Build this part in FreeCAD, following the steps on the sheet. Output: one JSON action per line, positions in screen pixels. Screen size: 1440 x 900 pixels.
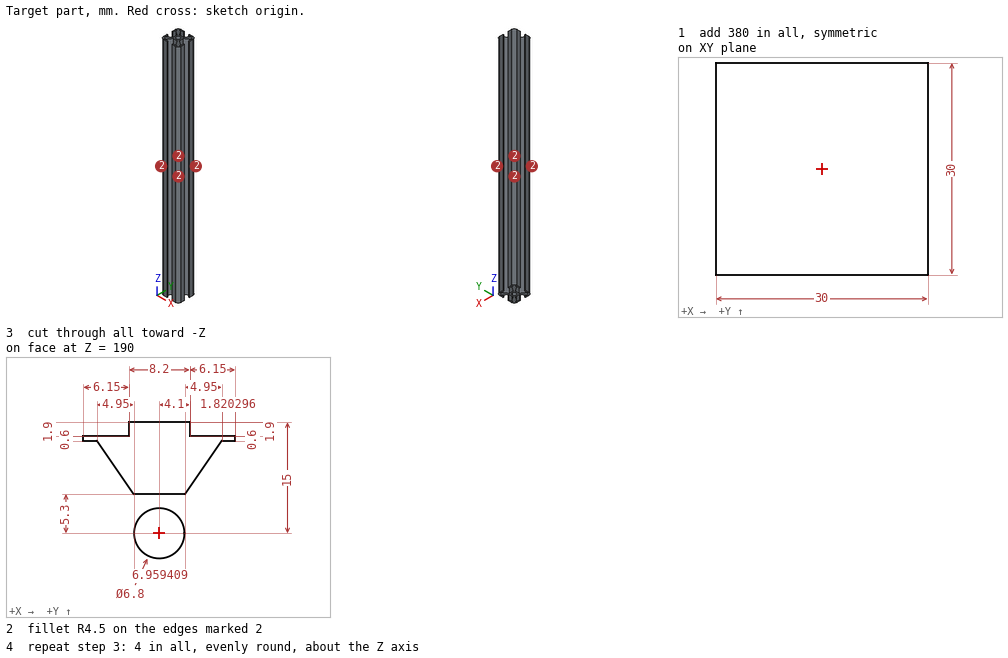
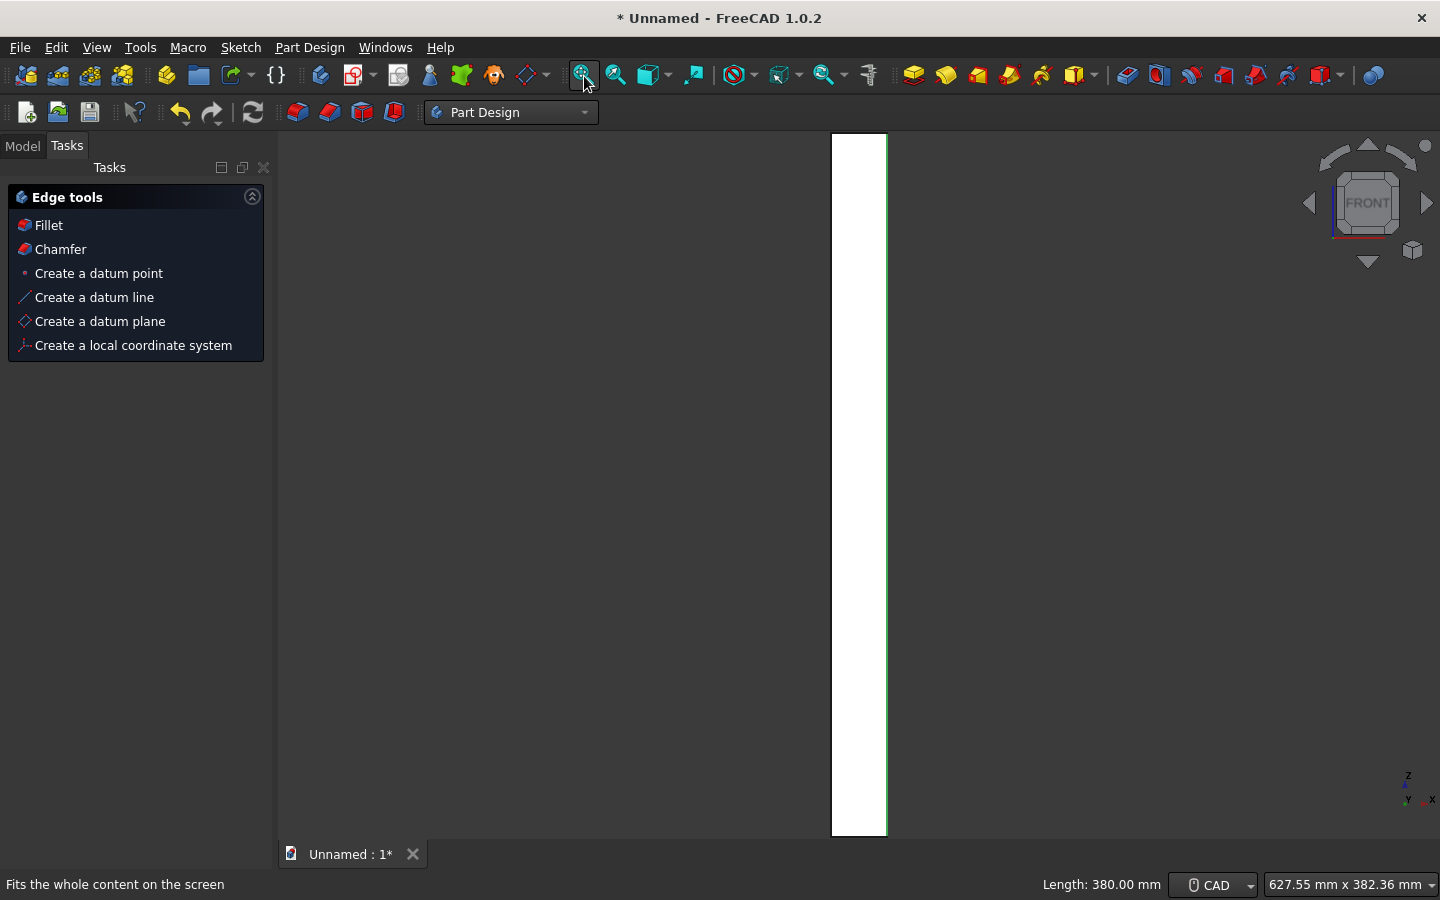
{"action": "left_click", "coordinate": [831, 484], "text": "ctrl"}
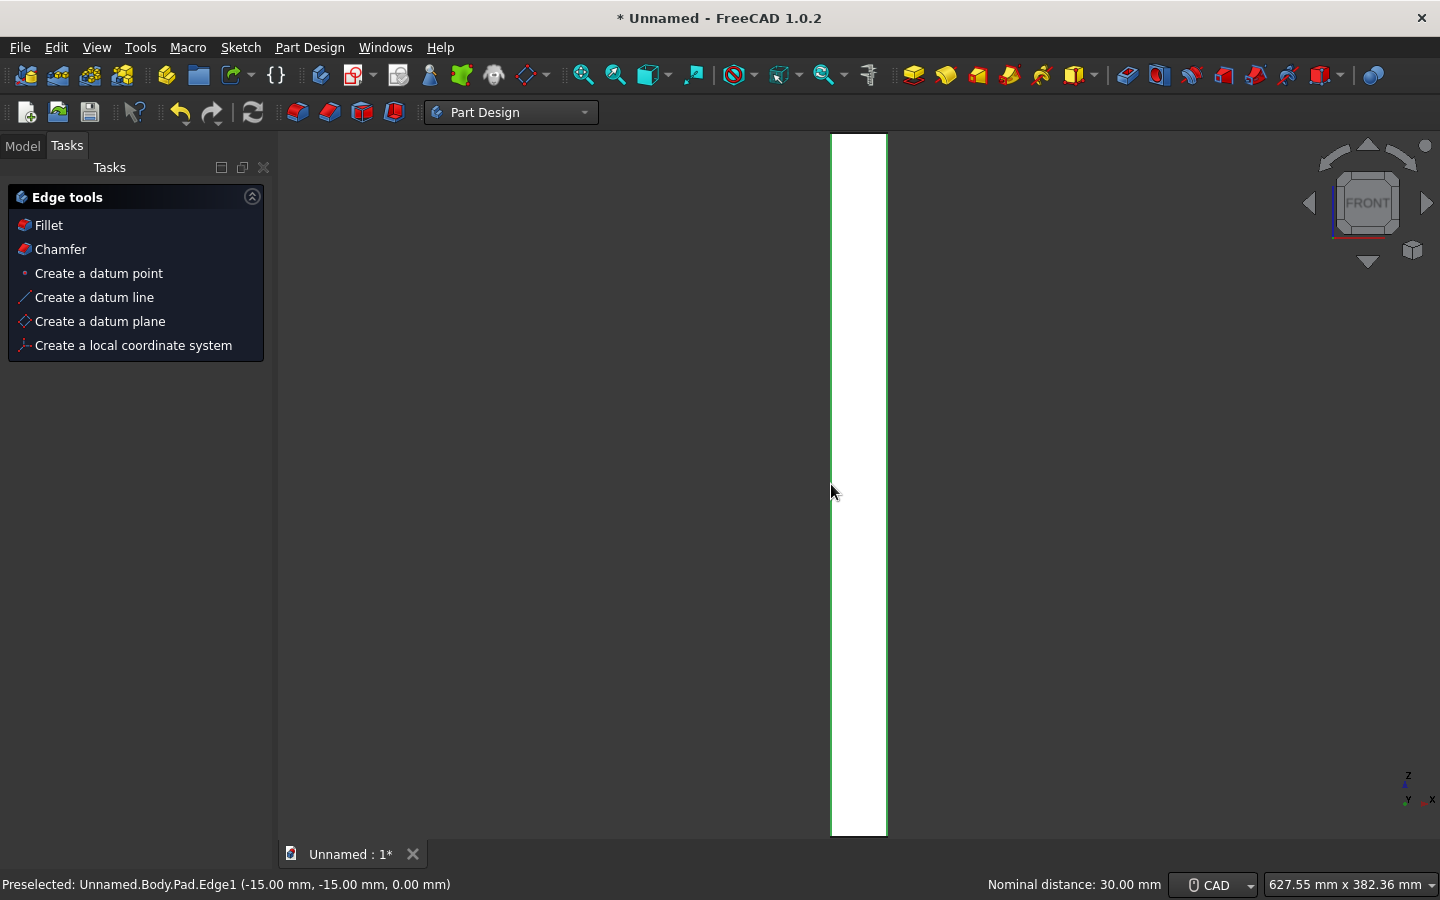
{"action": "key", "text": "3"}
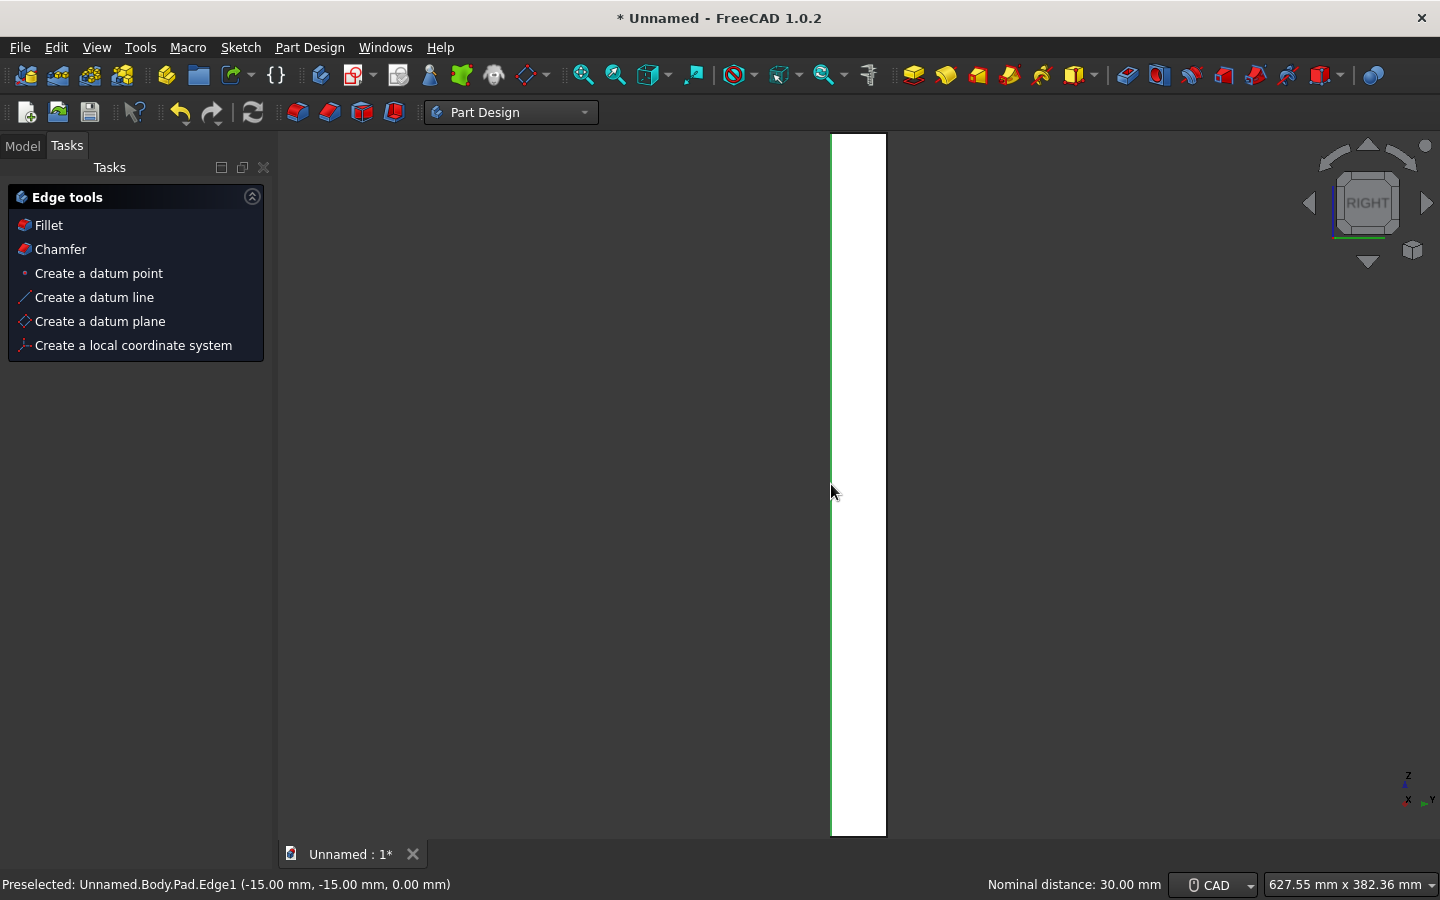
{"action": "left_click", "coordinate": [887, 484], "text": "ctrl"}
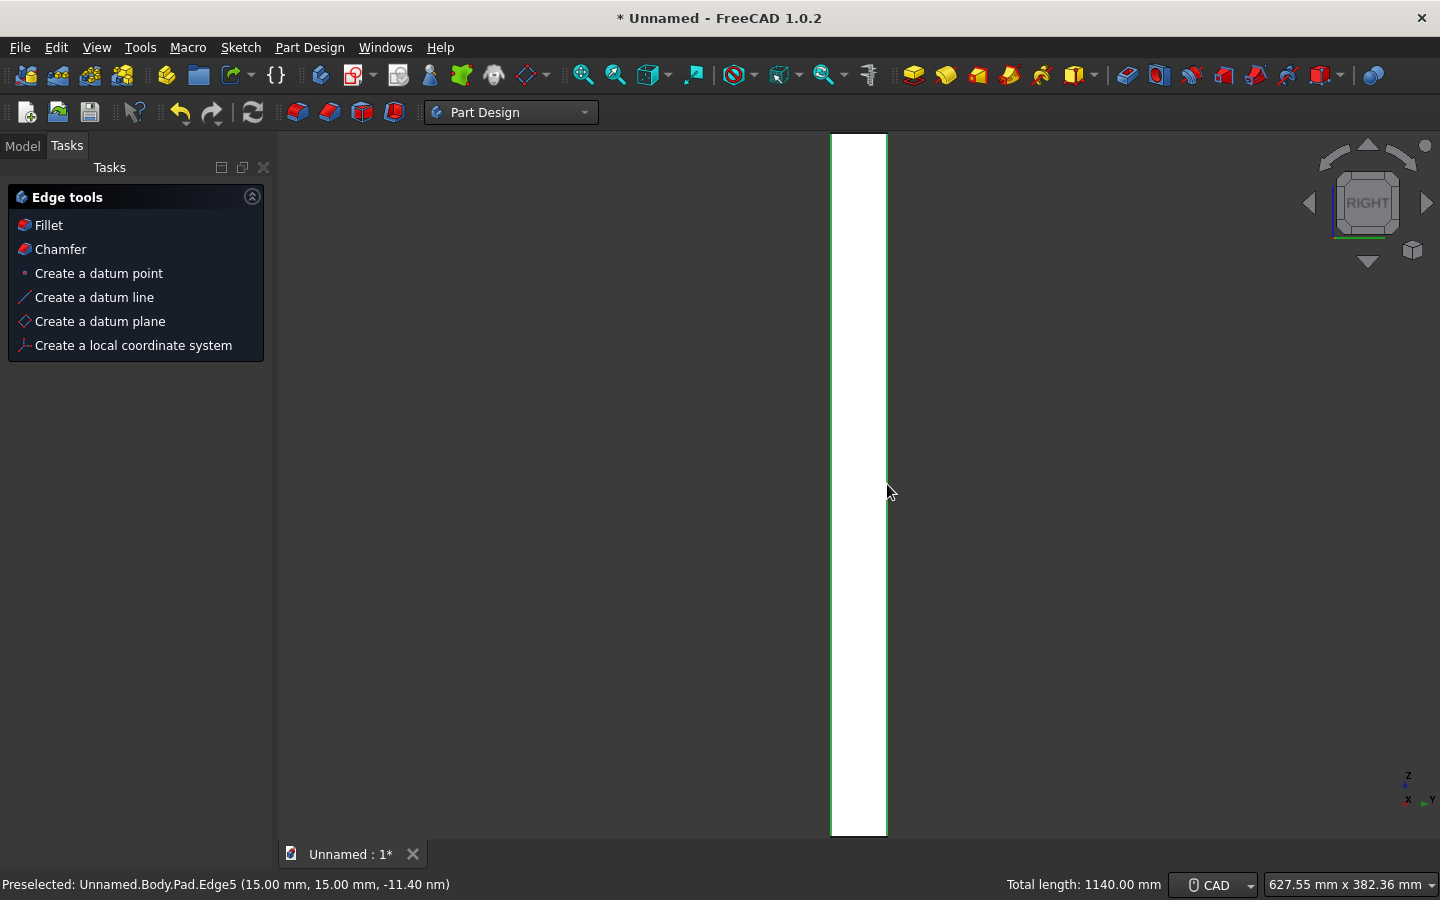
{"action": "key", "text": "5"}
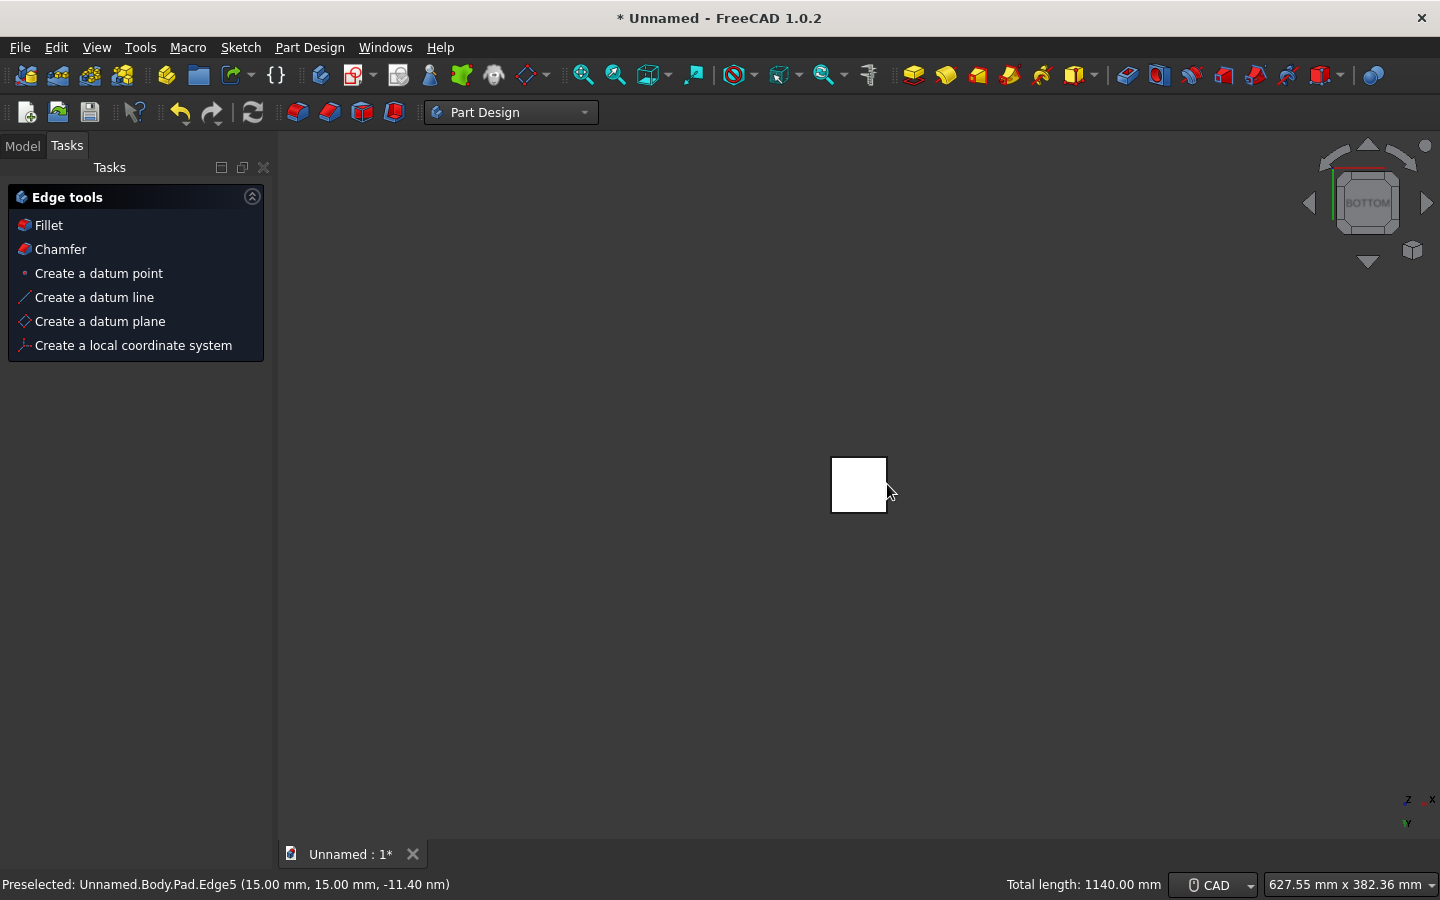
{"action": "left_click", "coordinate": [584, 76]}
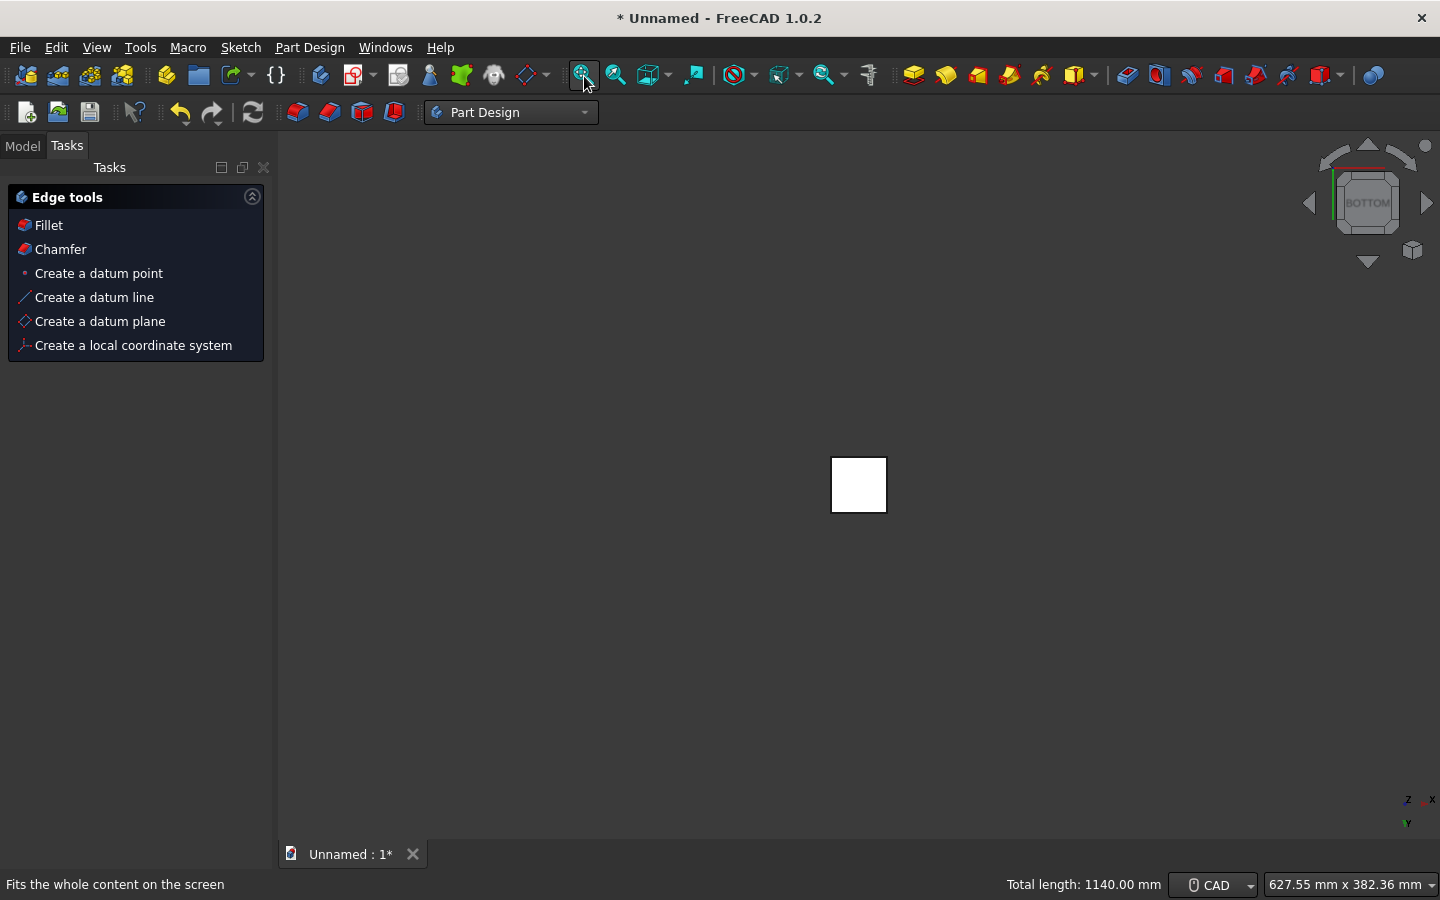
{"action": "key", "text": "4"}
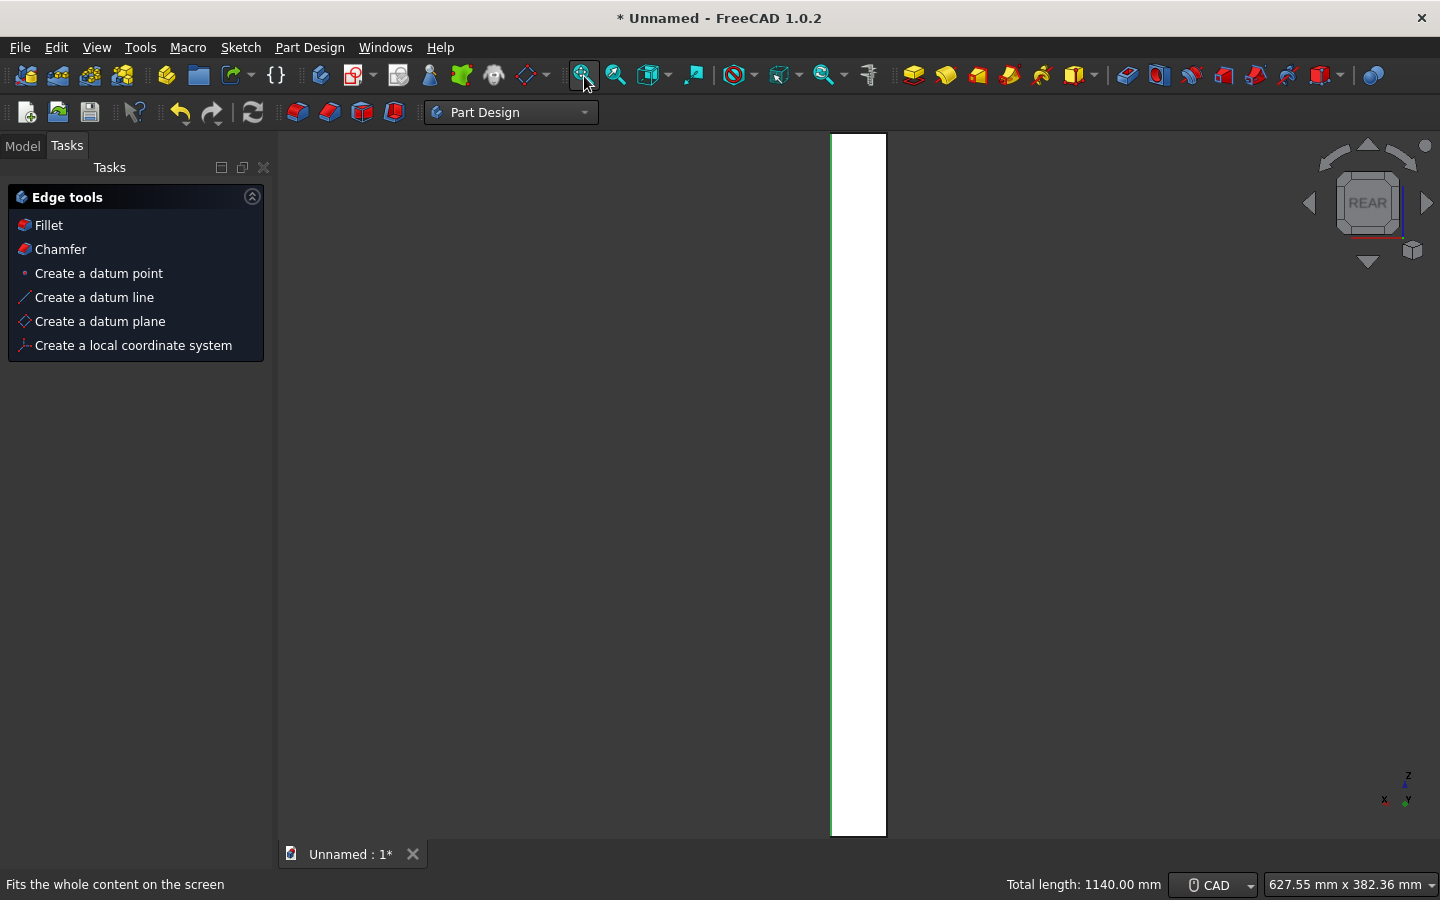
{"action": "left_click", "coordinate": [887, 484], "text": "ctrl"}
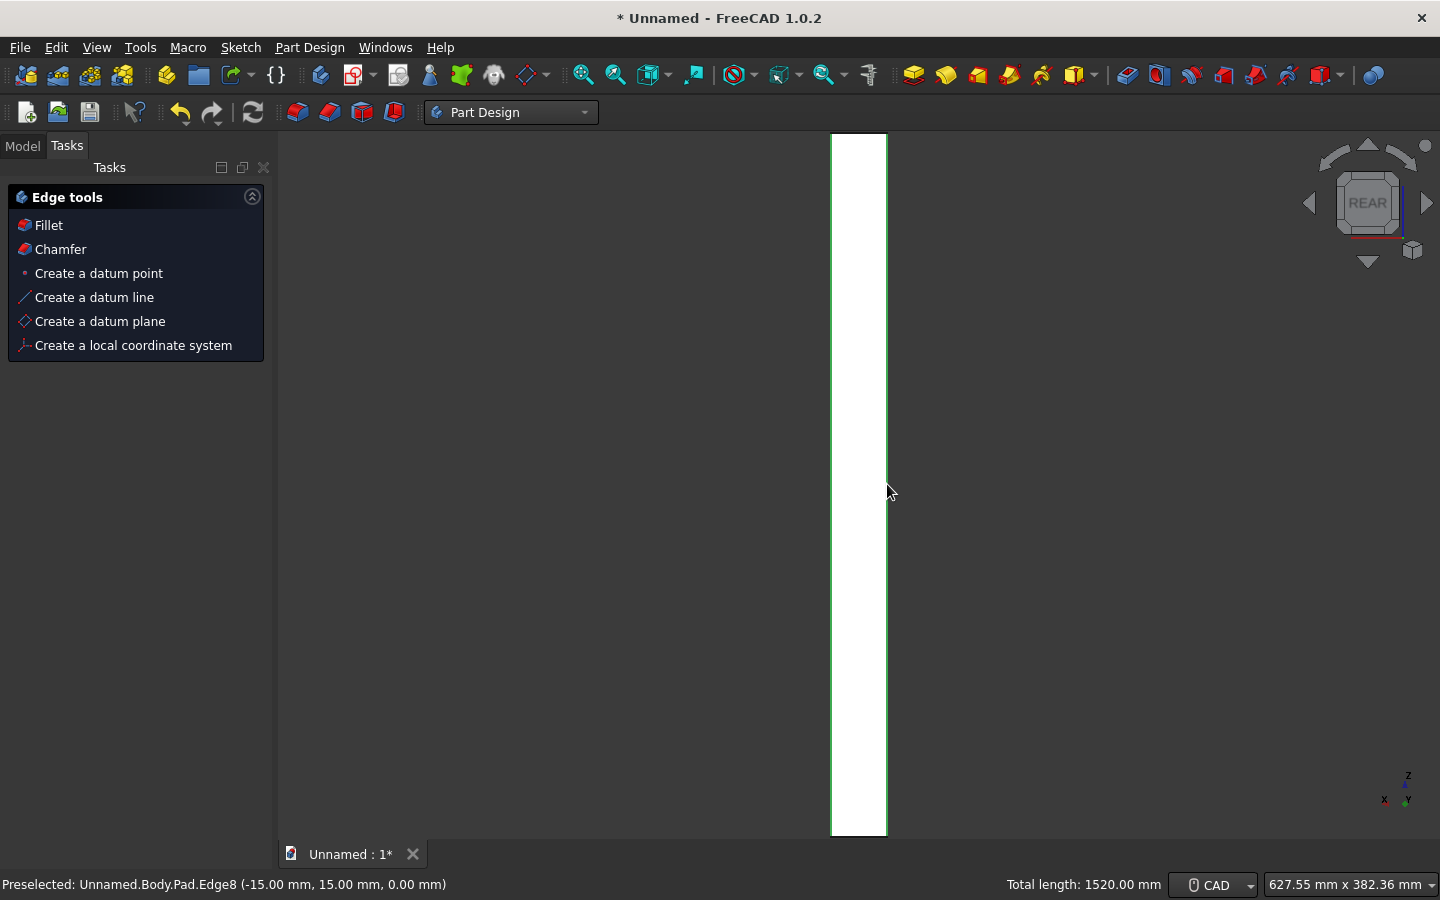
{"action": "left_click", "coordinate": [298, 112]}